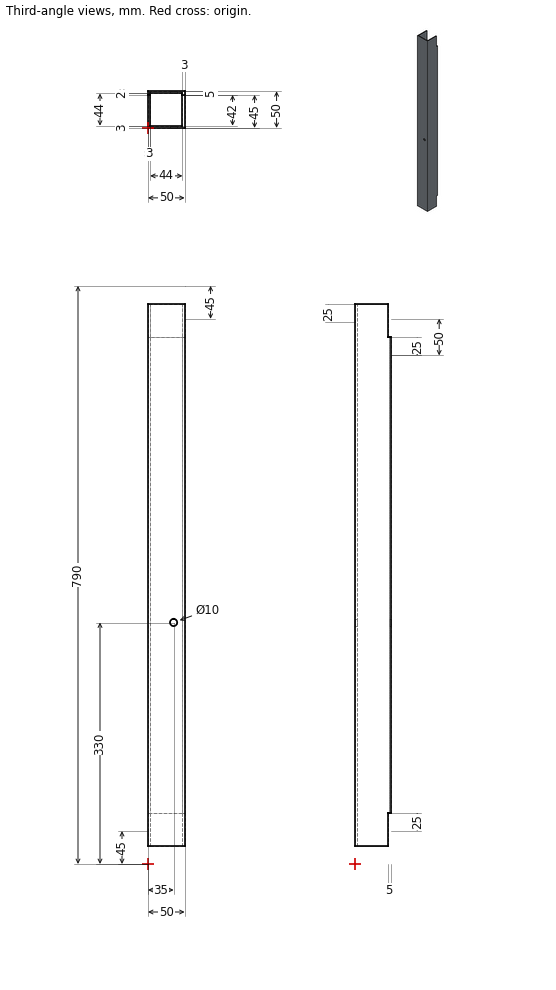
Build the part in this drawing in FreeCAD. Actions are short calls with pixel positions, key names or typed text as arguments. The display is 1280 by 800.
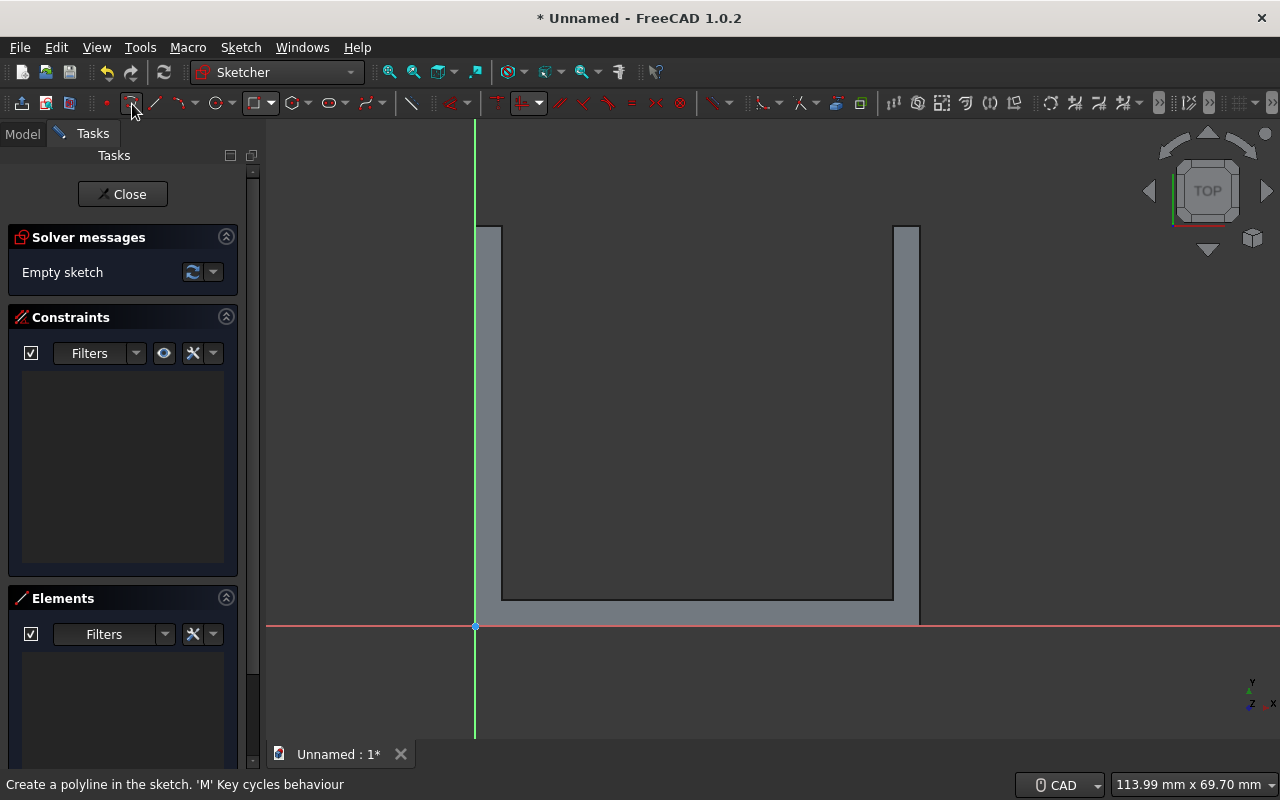
click(475, 626)
click(484, 226)
click(502, 226)
click(502, 600)
click(893, 600)
click(893, 226)
click(920, 226)
click(920, 617)
click(475, 626)
key(Escape)
key(Escape)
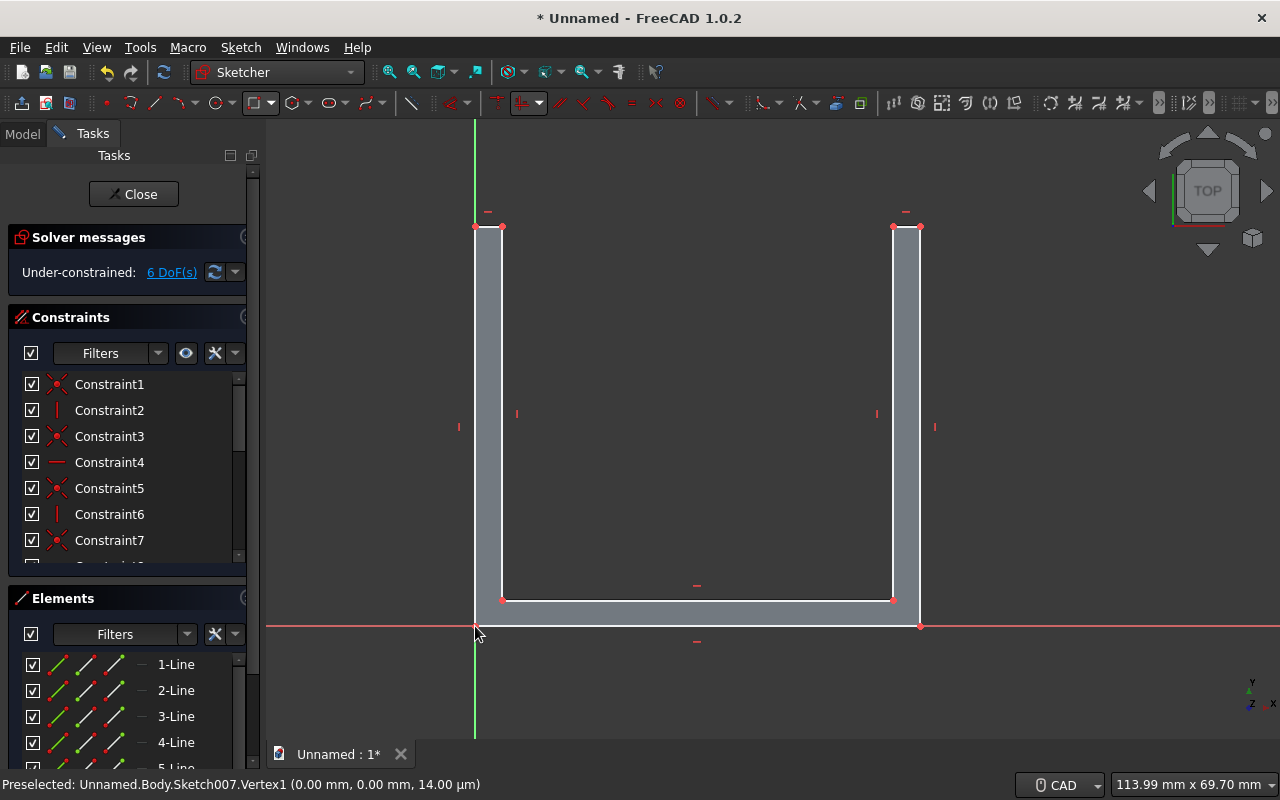
click(450, 104)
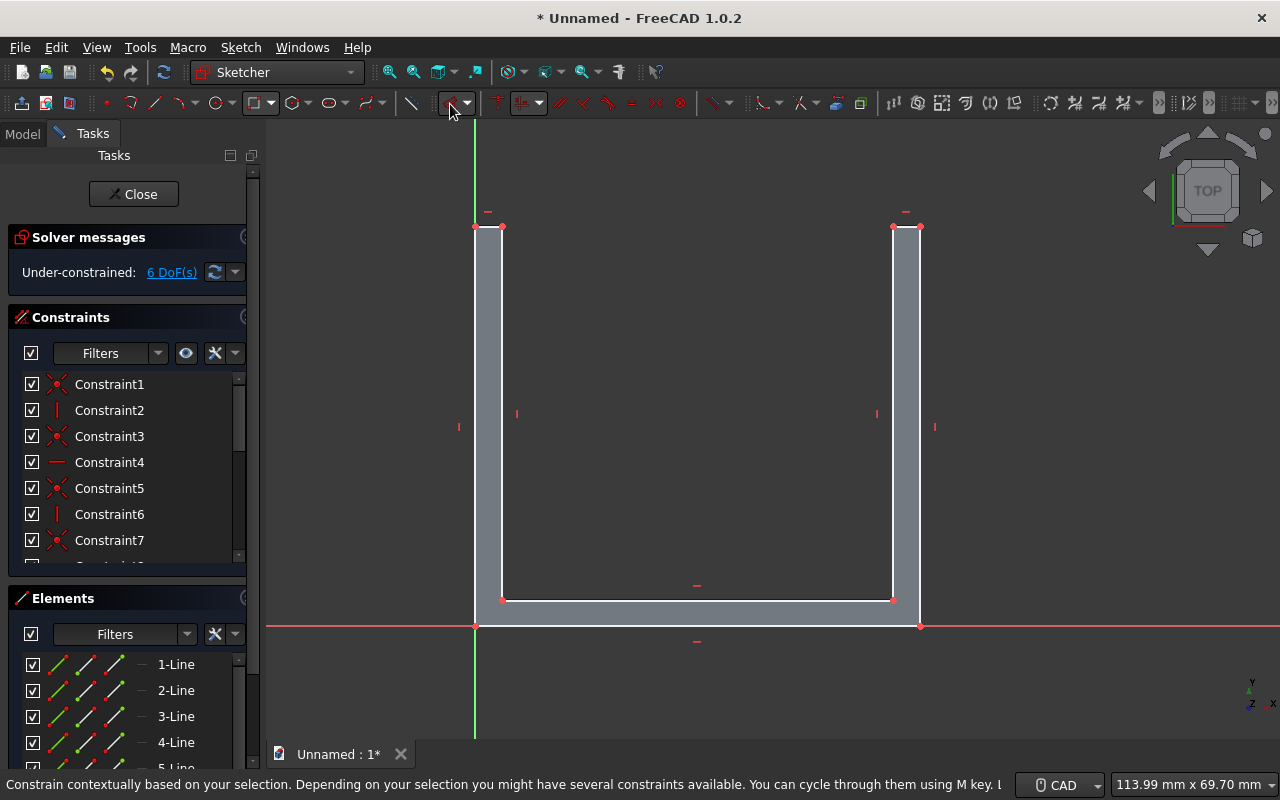
scroll(486, 227, up, 2)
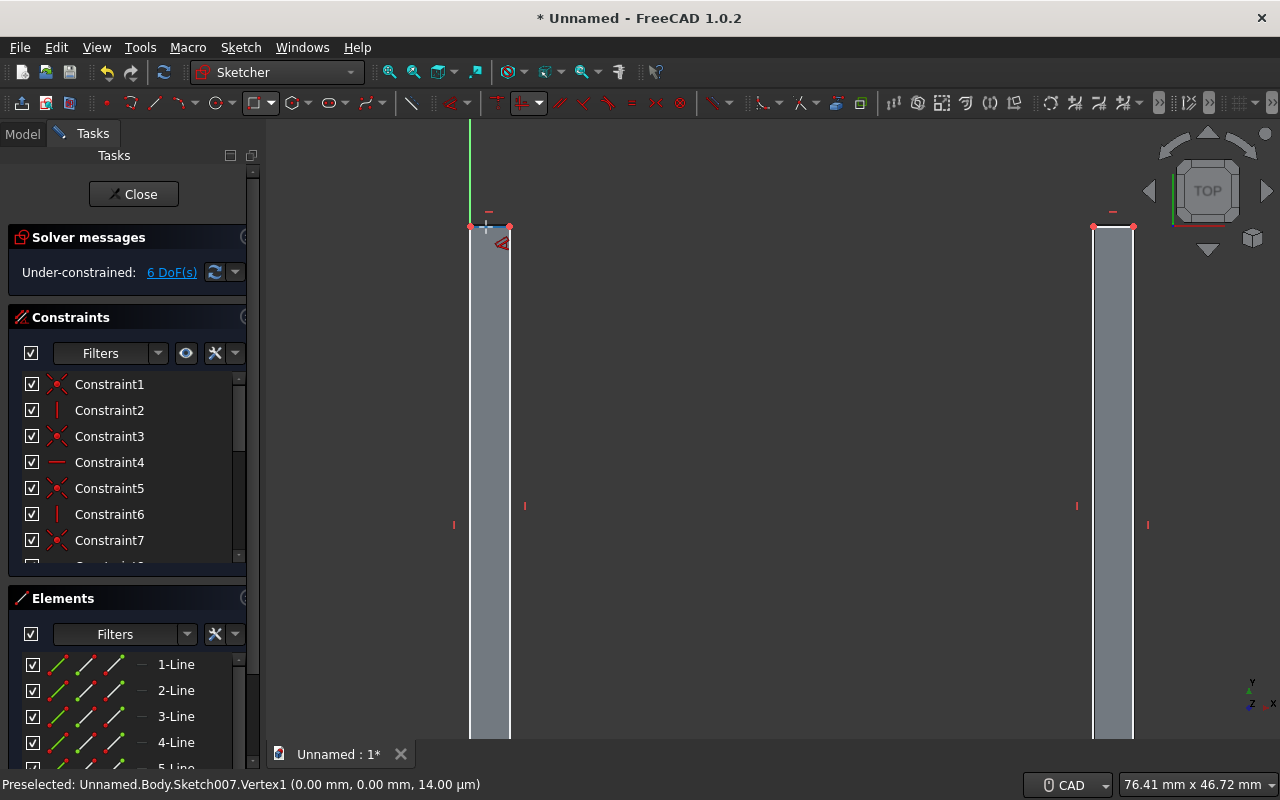
click(486, 227)
click(490, 193)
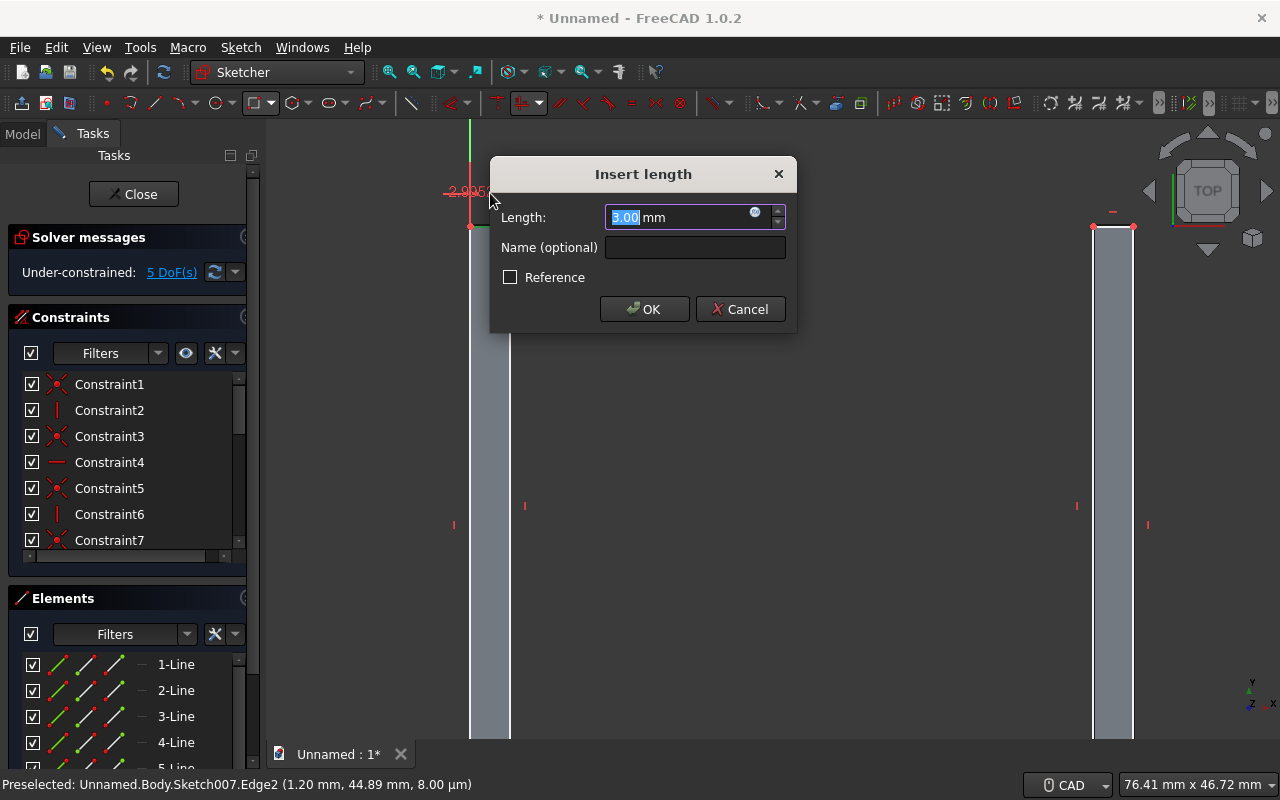
text(3)
key(Return)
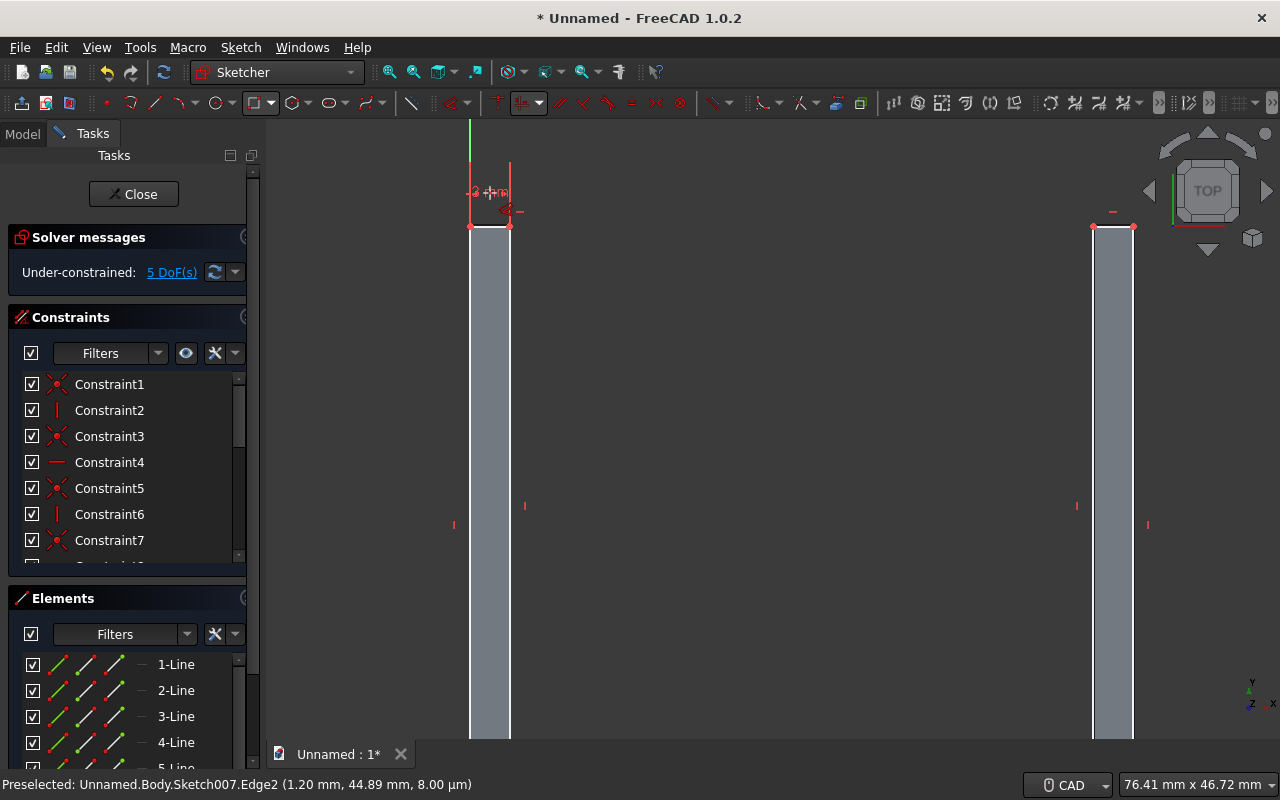
click(1105, 227)
click(1104, 193)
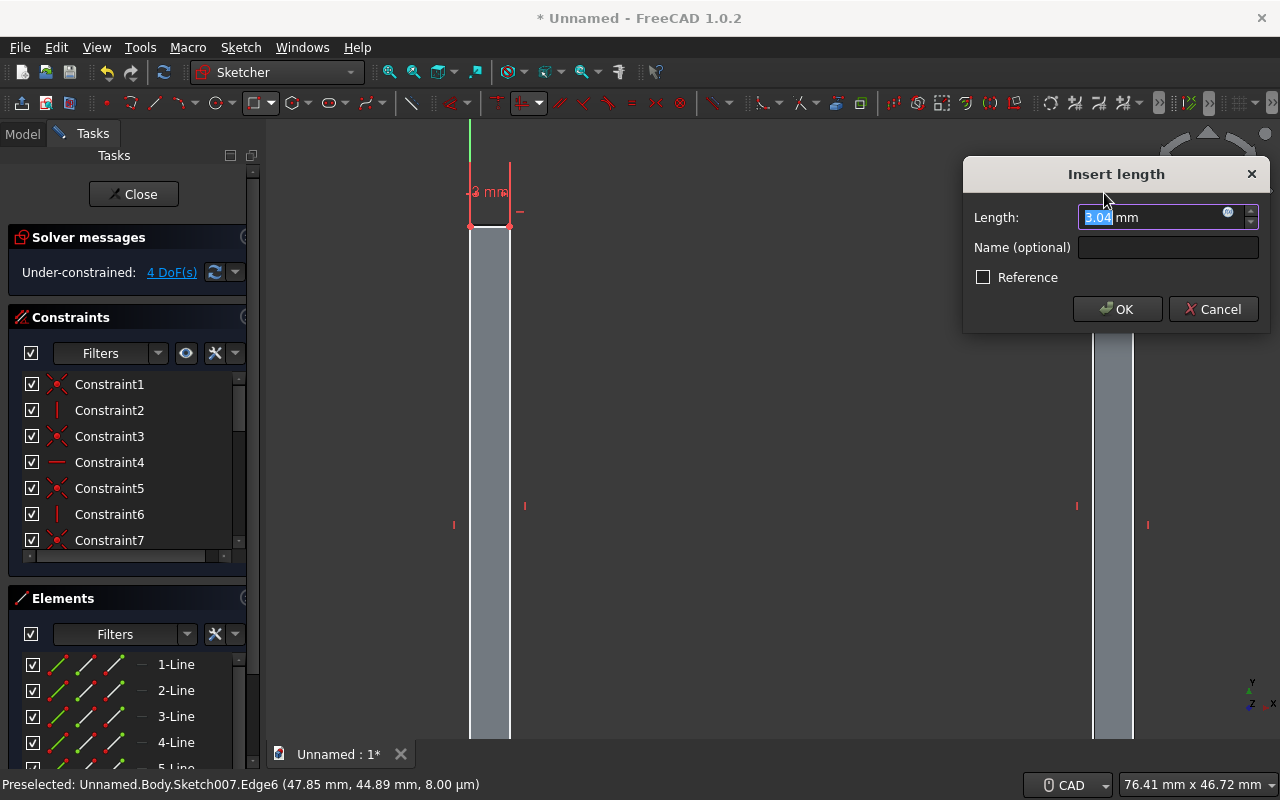
text(3)
key(Return)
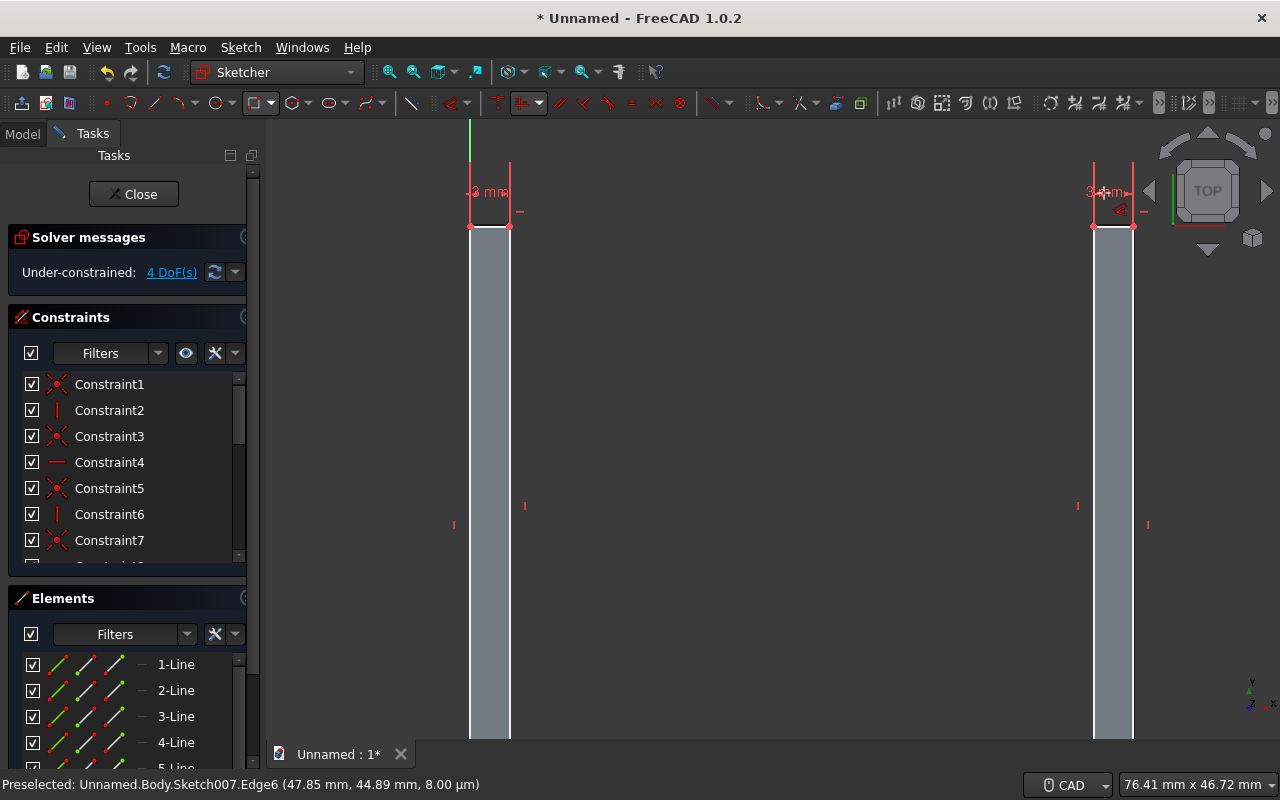
click(470, 644)
click(436, 469)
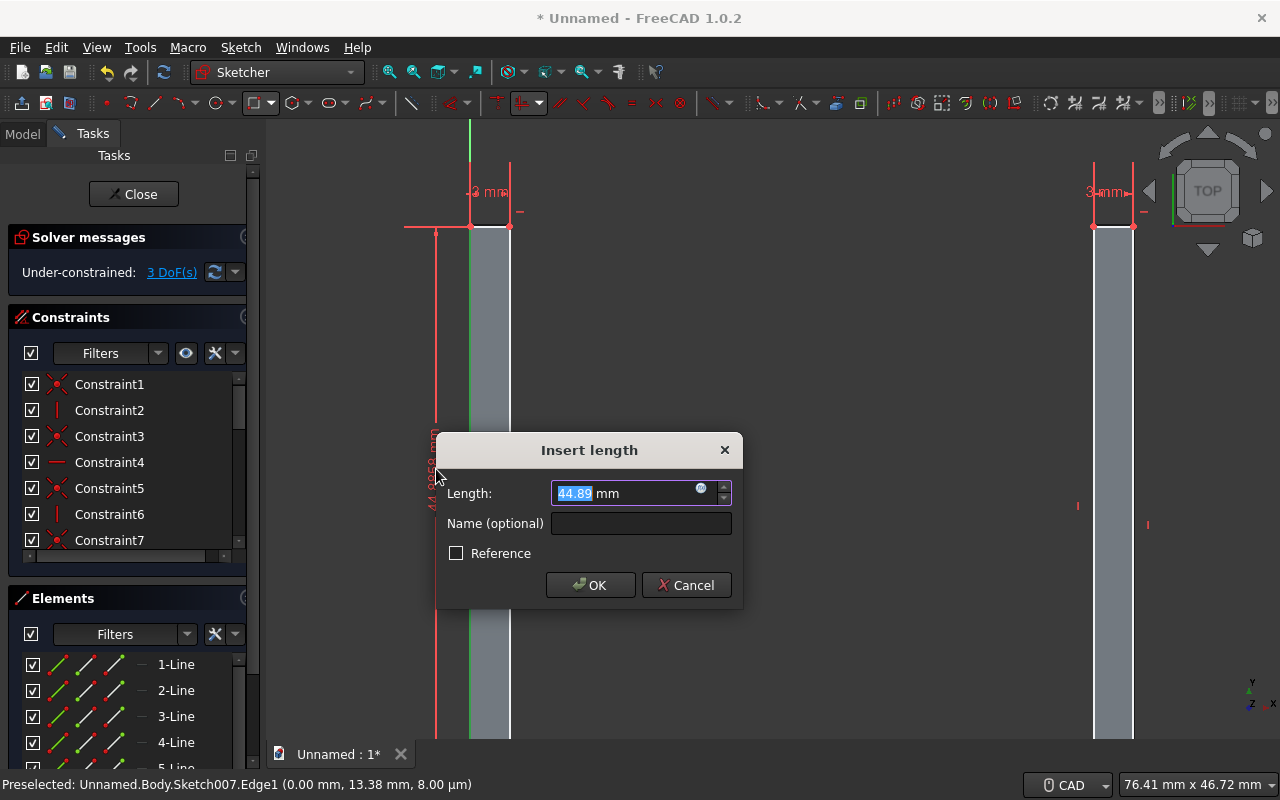
text(45)
key(Return)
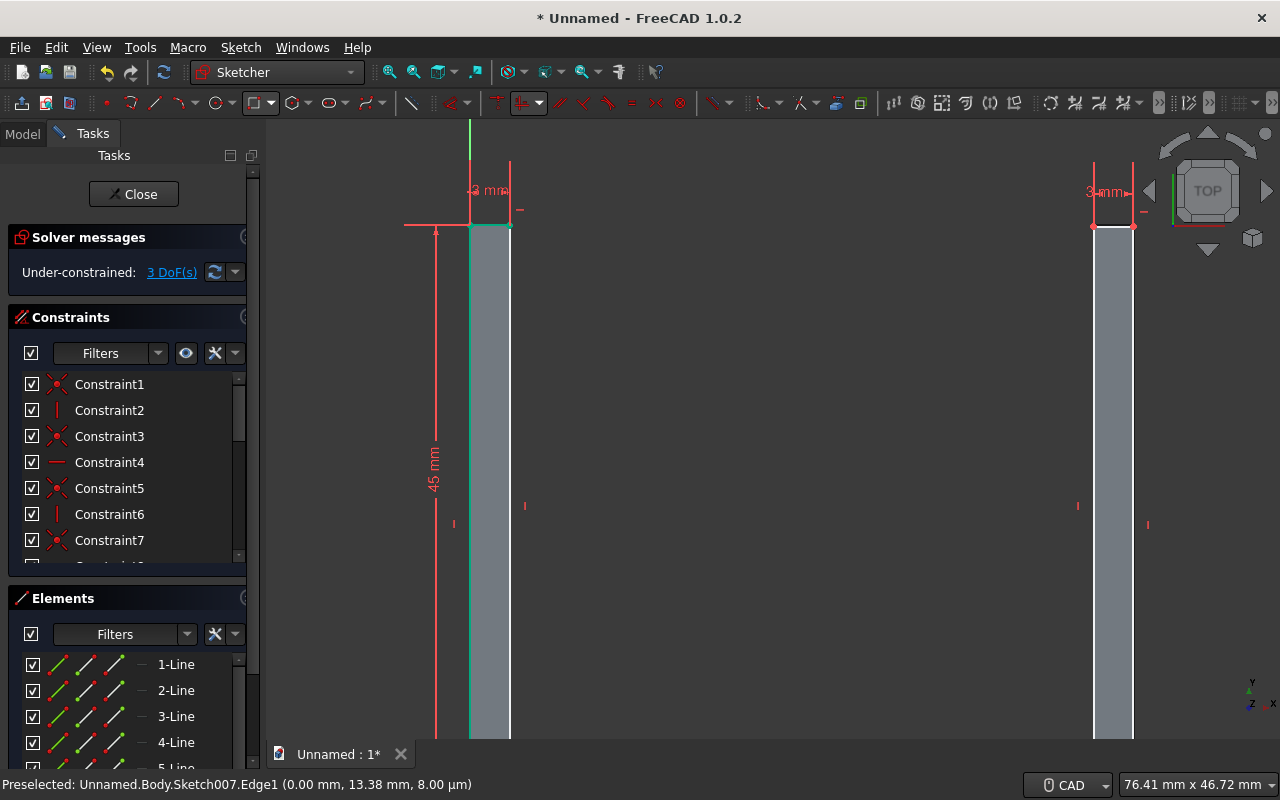
click(510, 393)
click(544, 468)